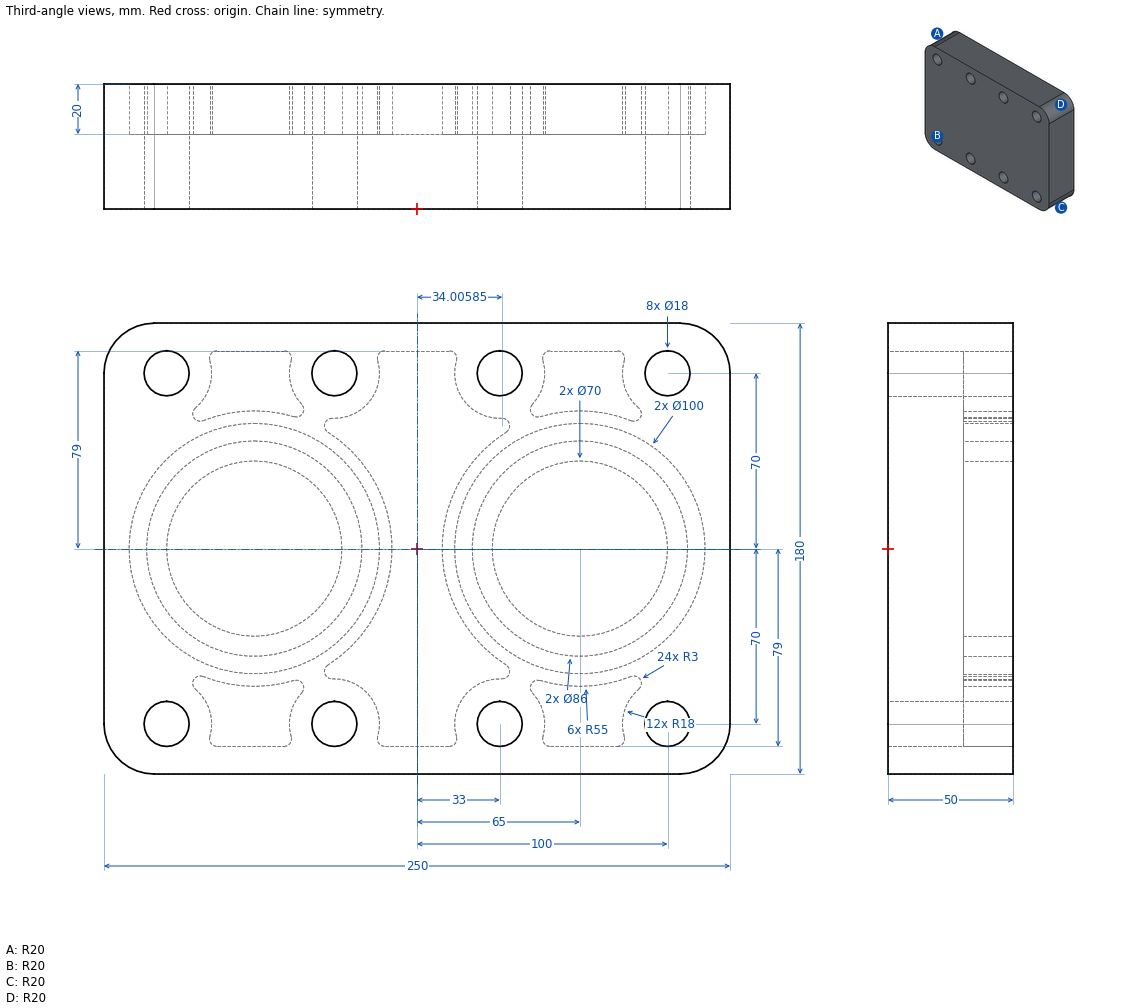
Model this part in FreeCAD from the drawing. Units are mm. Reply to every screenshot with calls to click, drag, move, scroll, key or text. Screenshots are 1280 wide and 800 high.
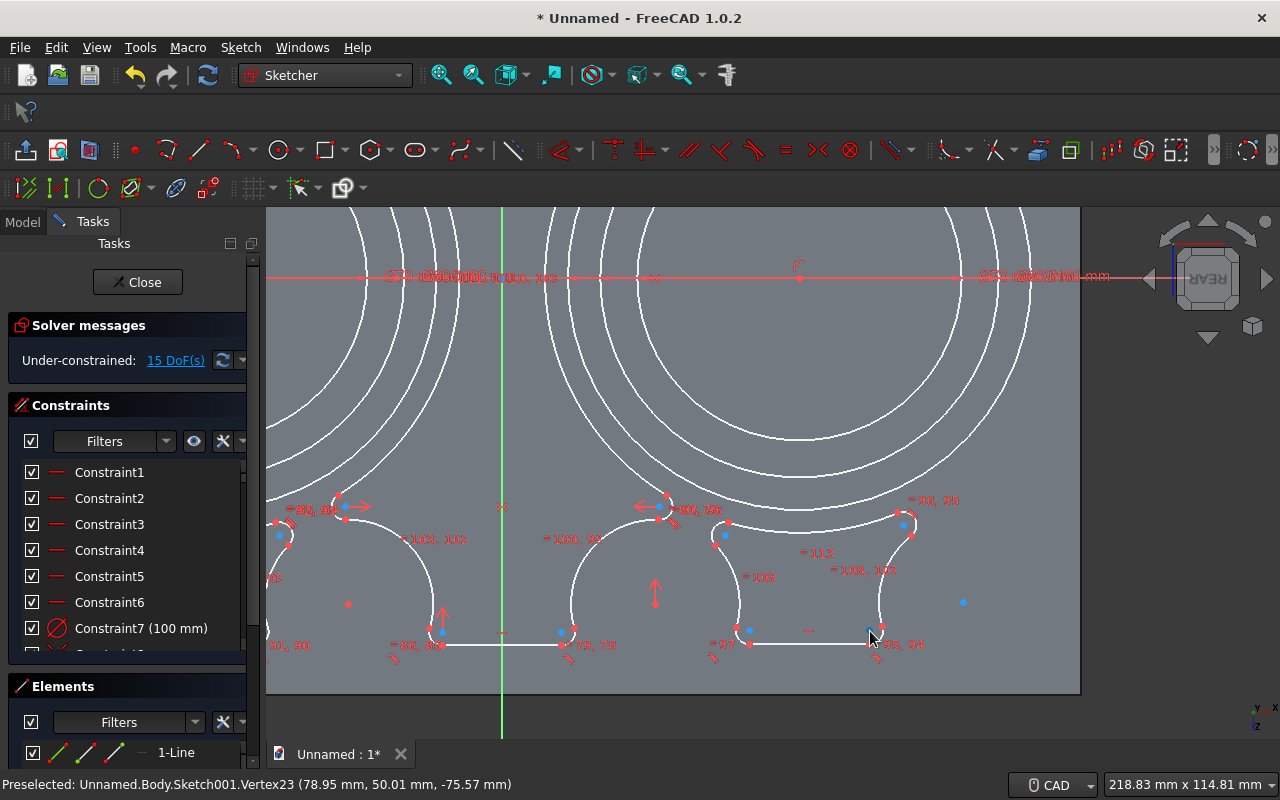
click(870, 631)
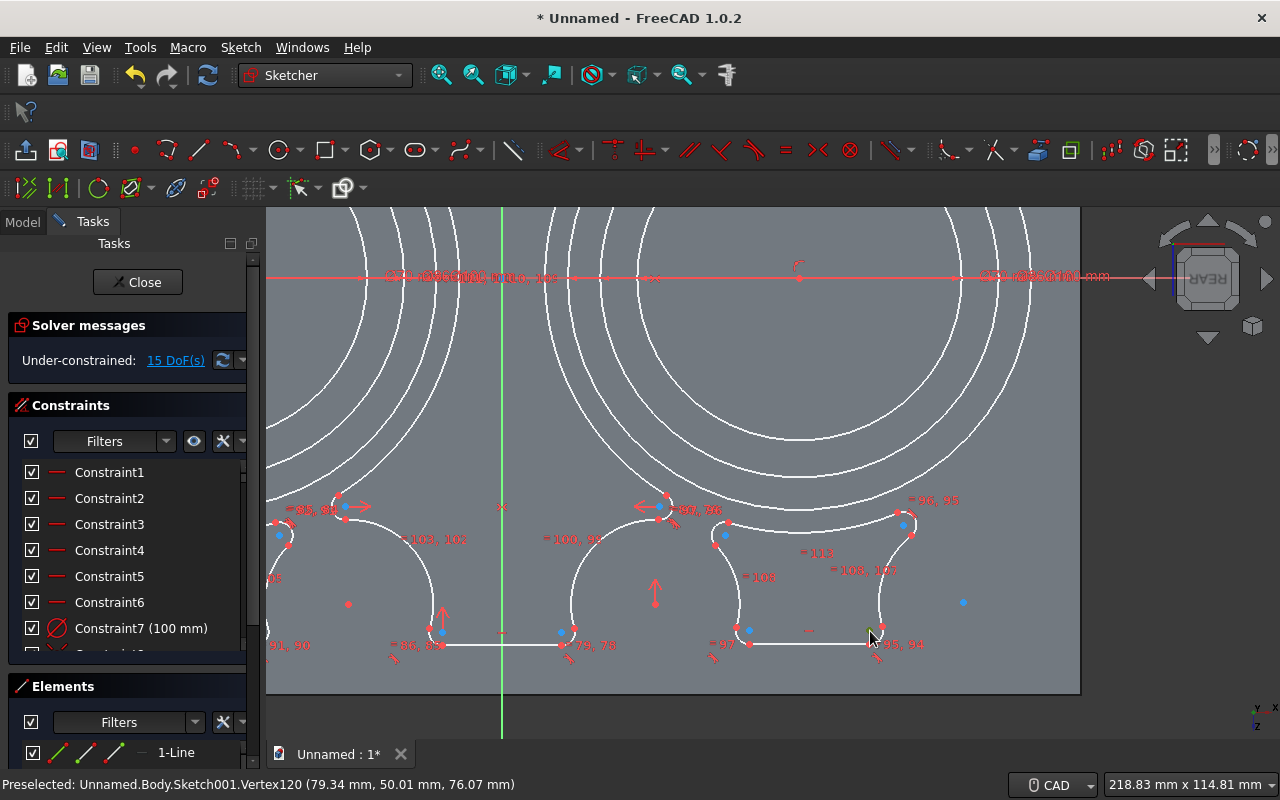
click(704, 278)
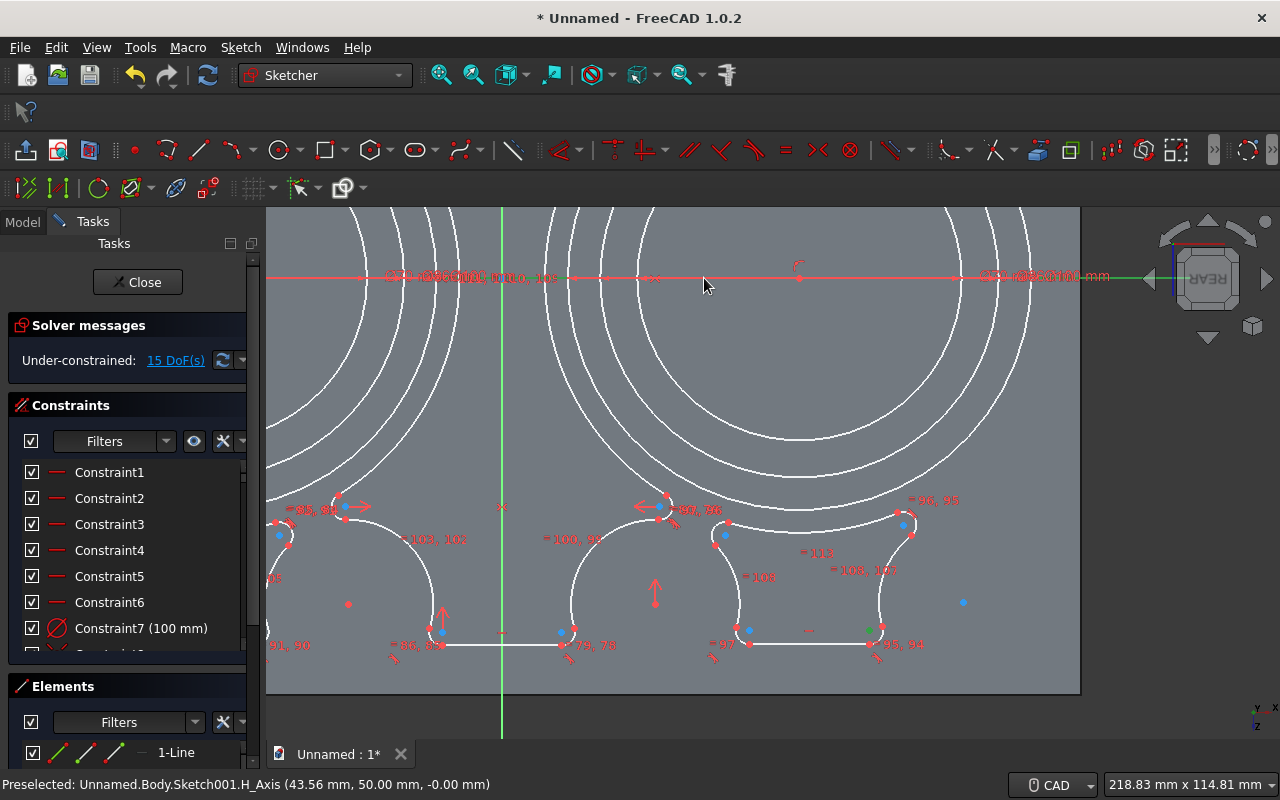
click(818, 150)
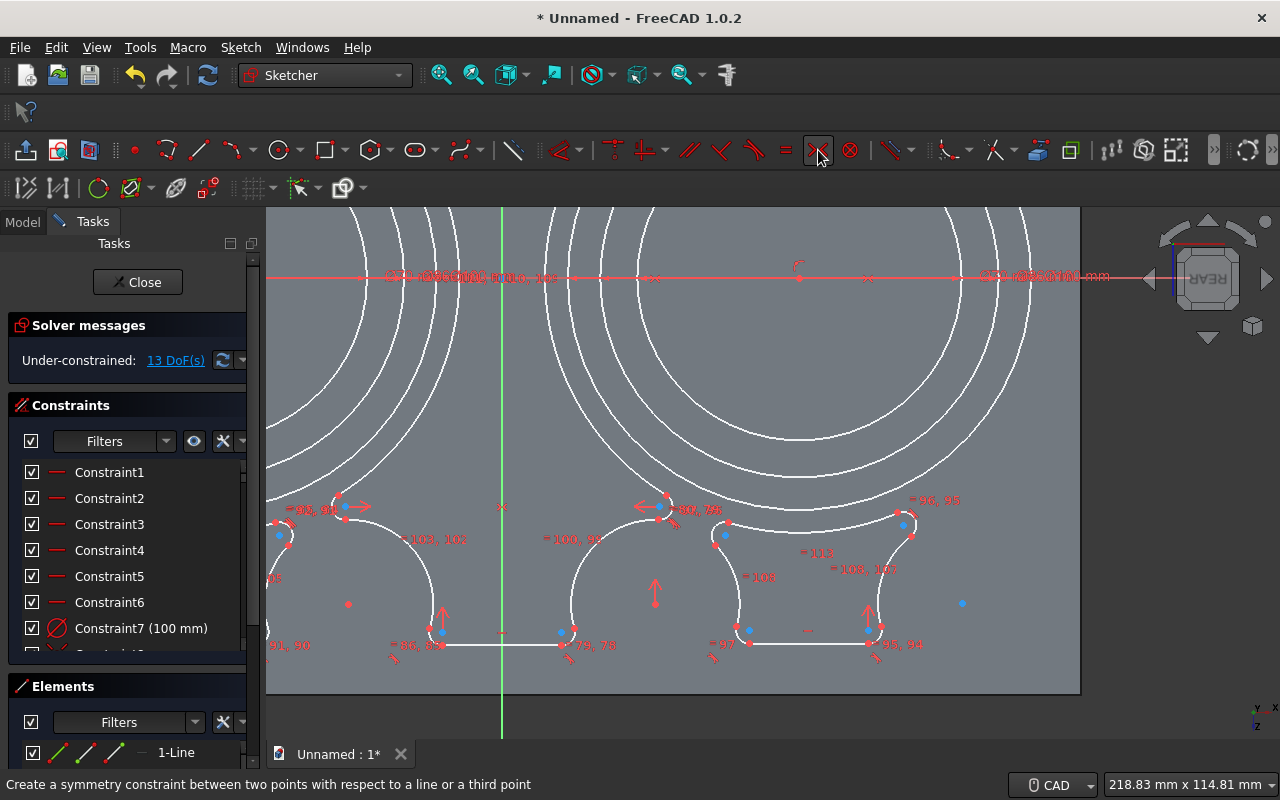
click(560, 150)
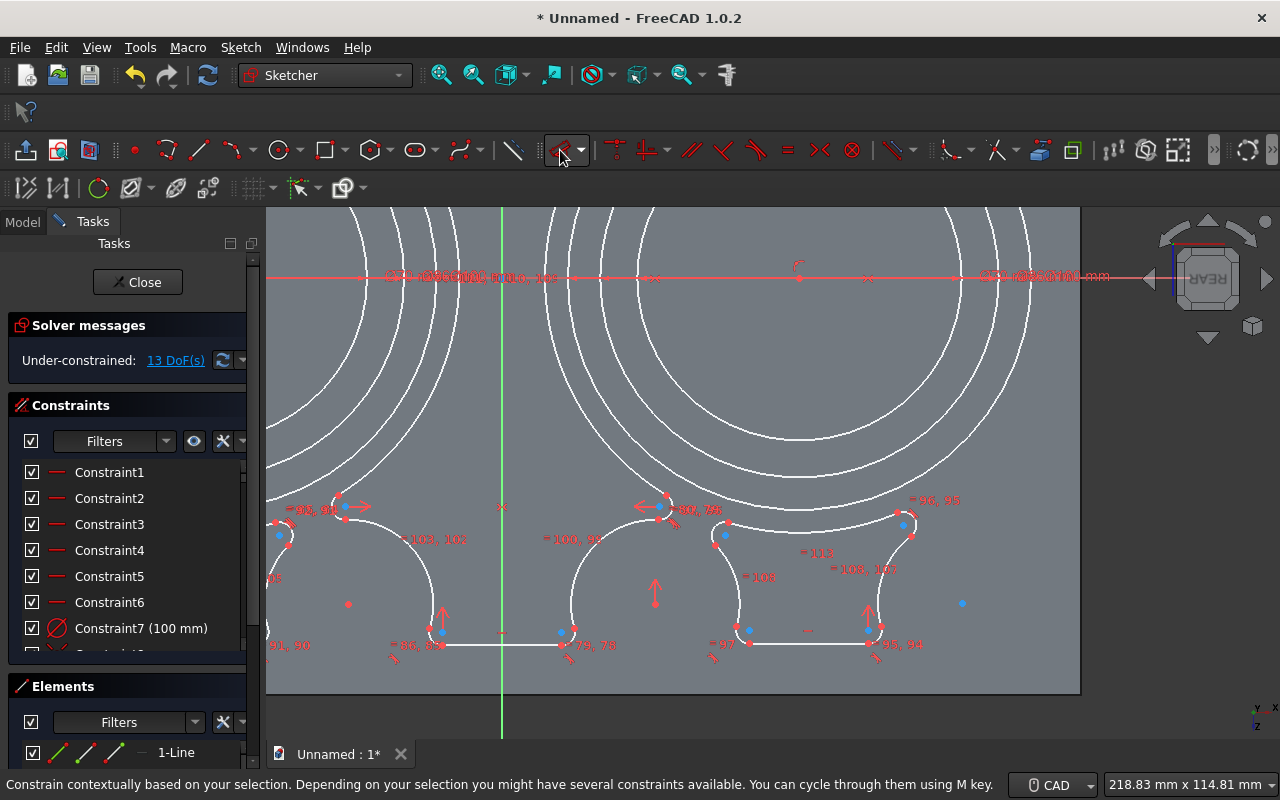
scroll(870, 632, down, 4)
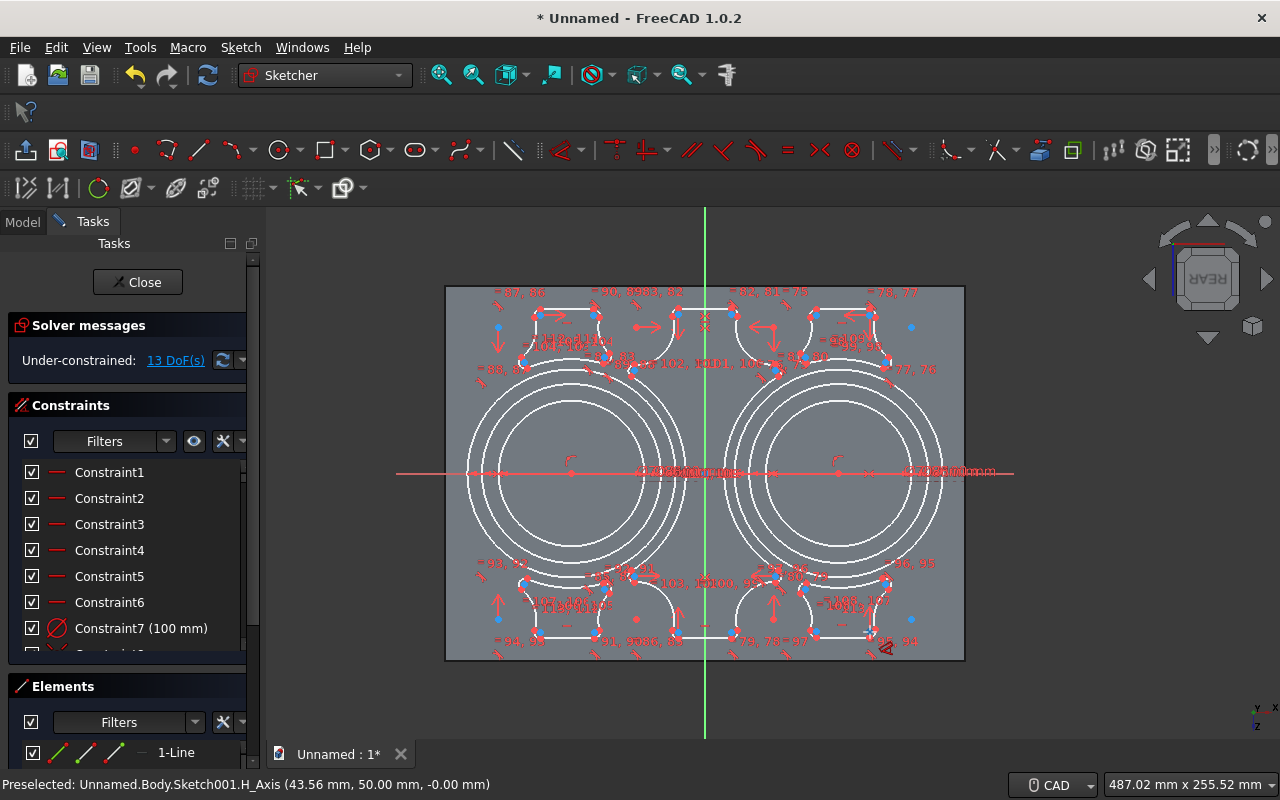
scroll(811, 312, up, 10)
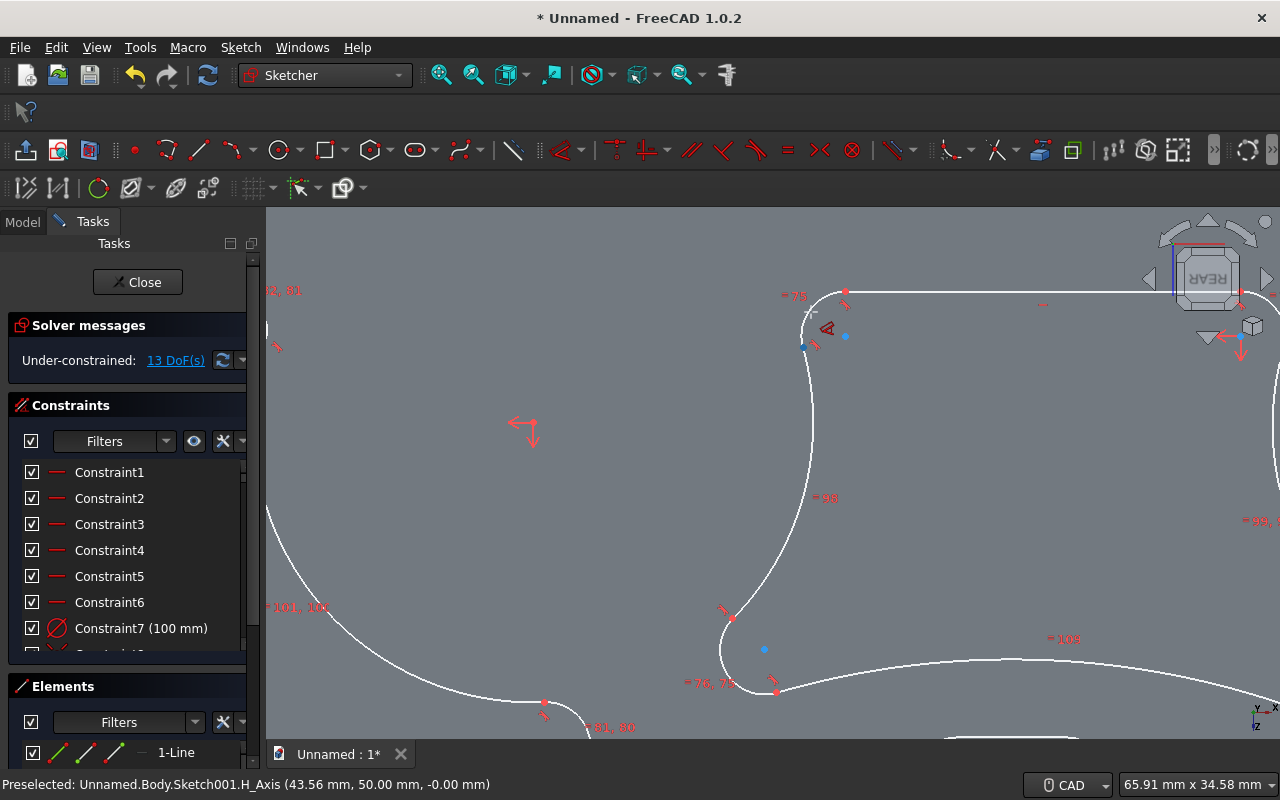
click(811, 309)
click(786, 289)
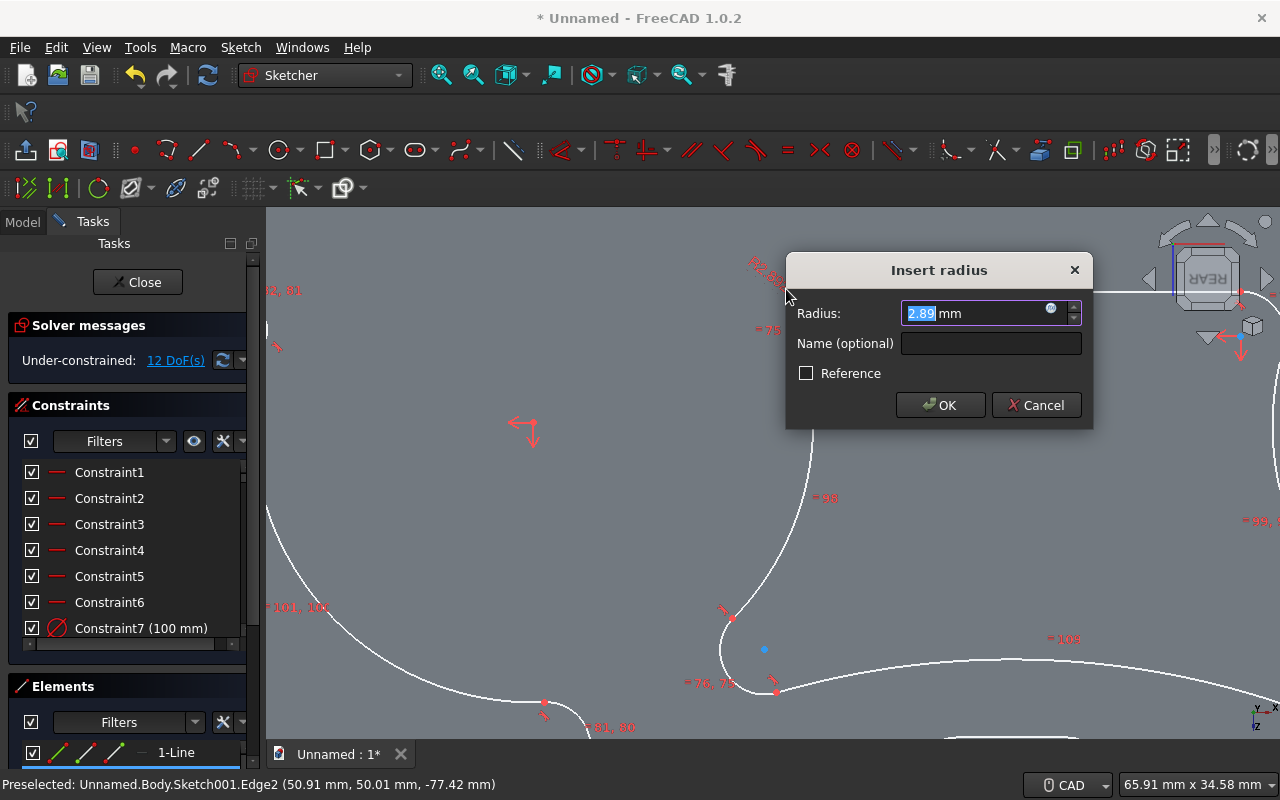
text(3)
key(Return)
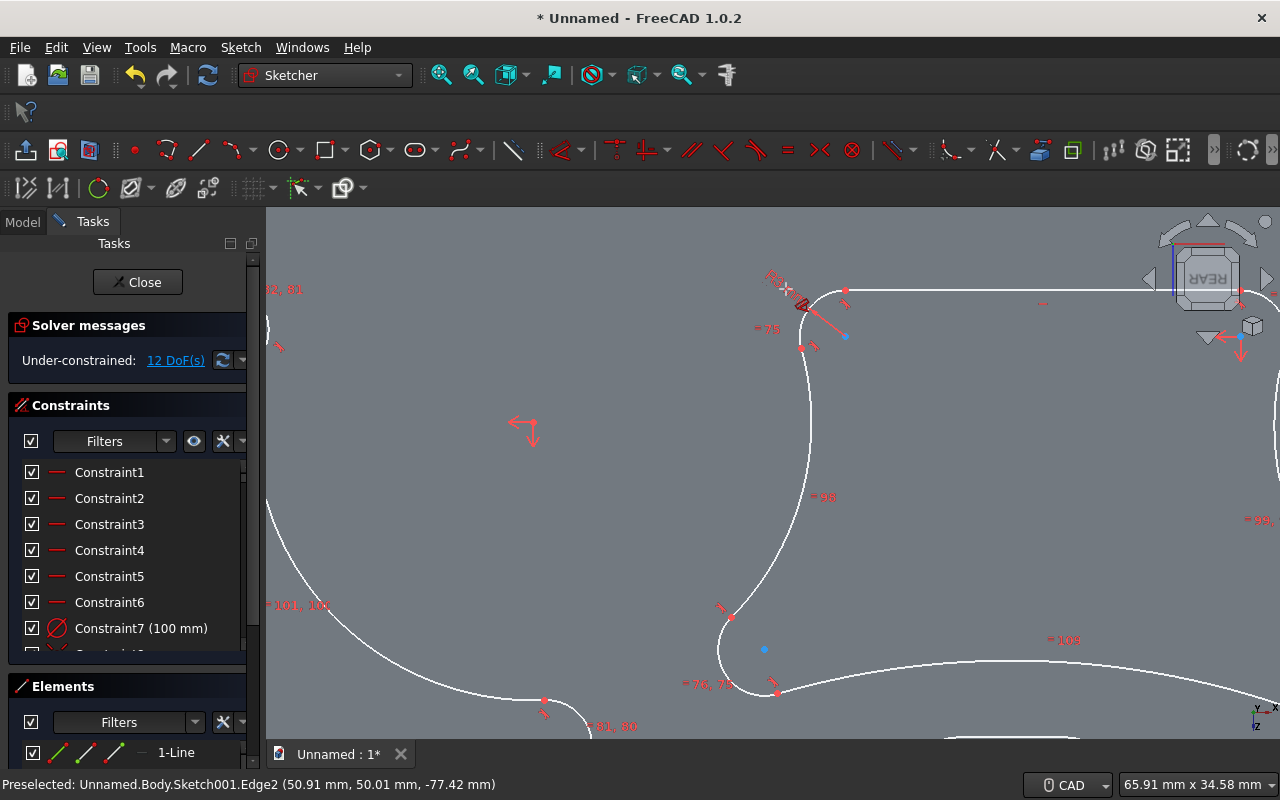
scroll(811, 312, down, 10)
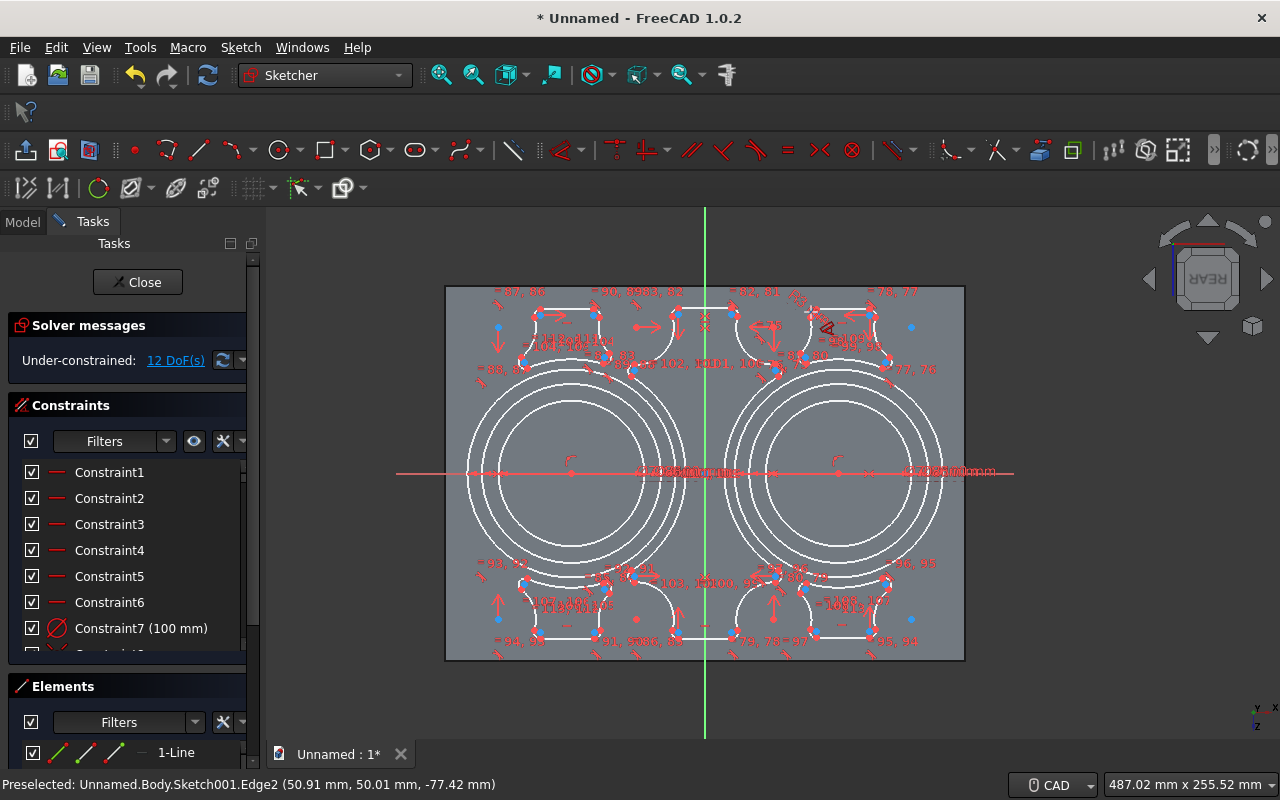
click(808, 344)
click(743, 390)